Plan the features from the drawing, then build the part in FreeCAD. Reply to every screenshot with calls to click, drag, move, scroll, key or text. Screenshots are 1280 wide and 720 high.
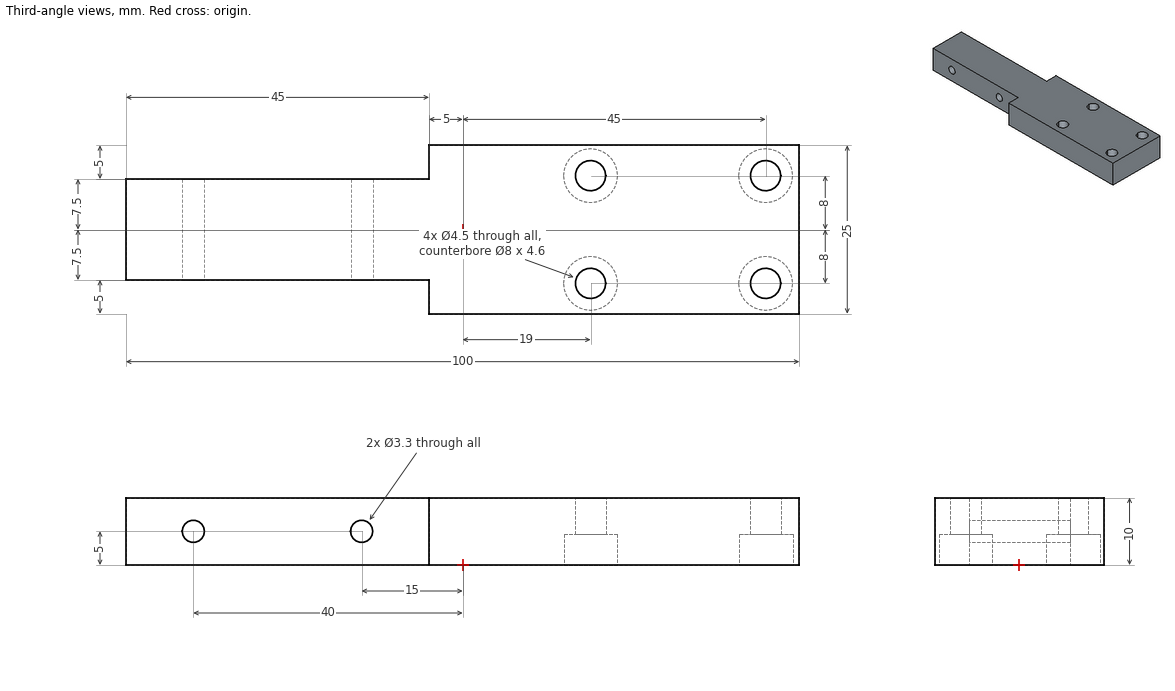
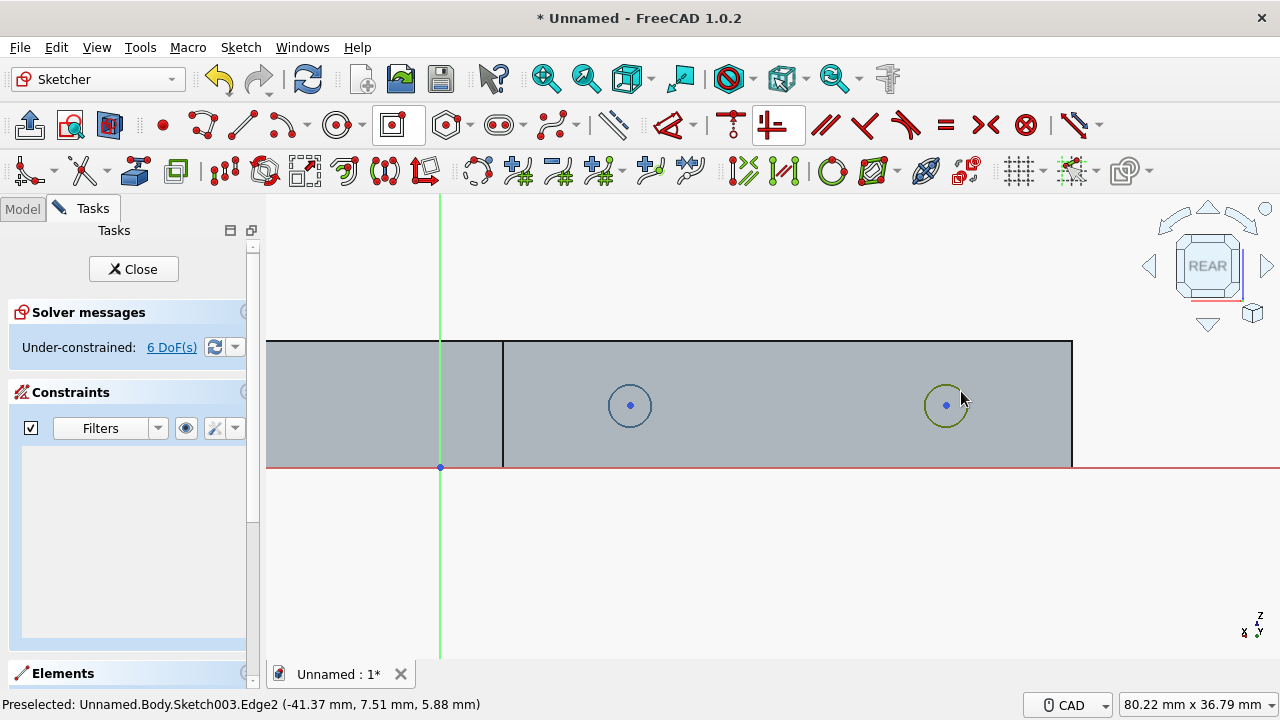
click(946, 126)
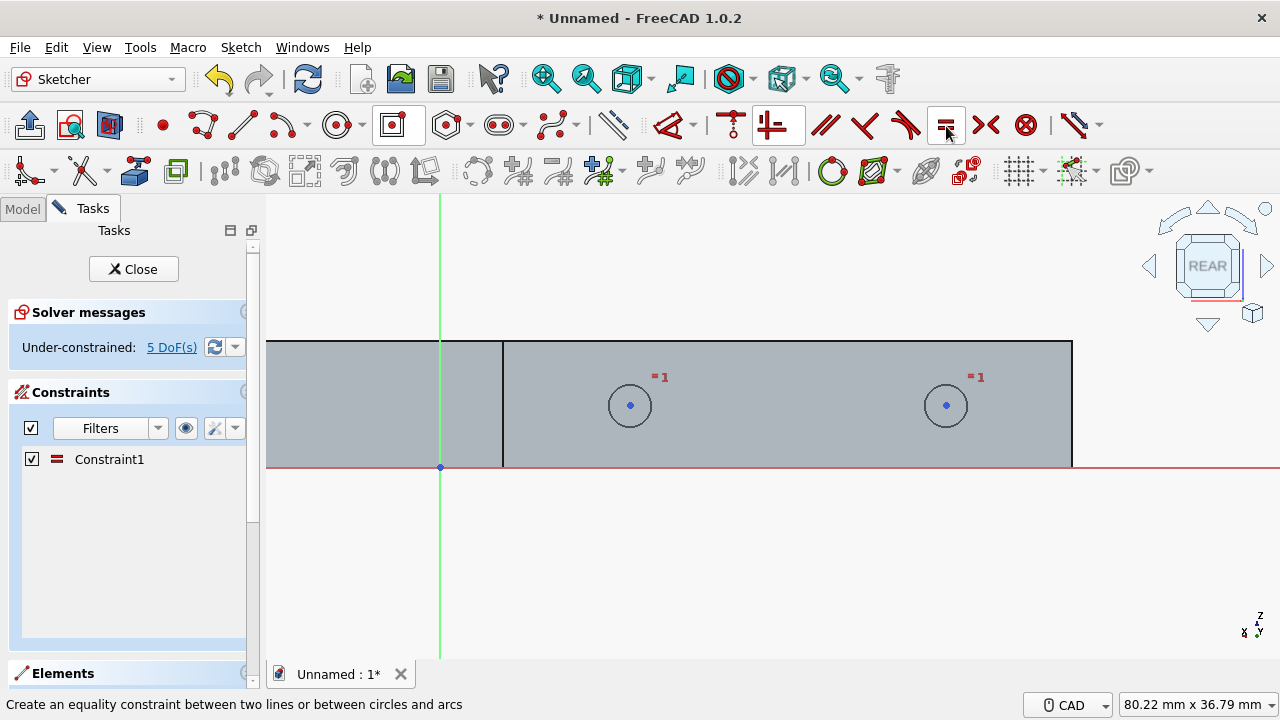
click(630, 406)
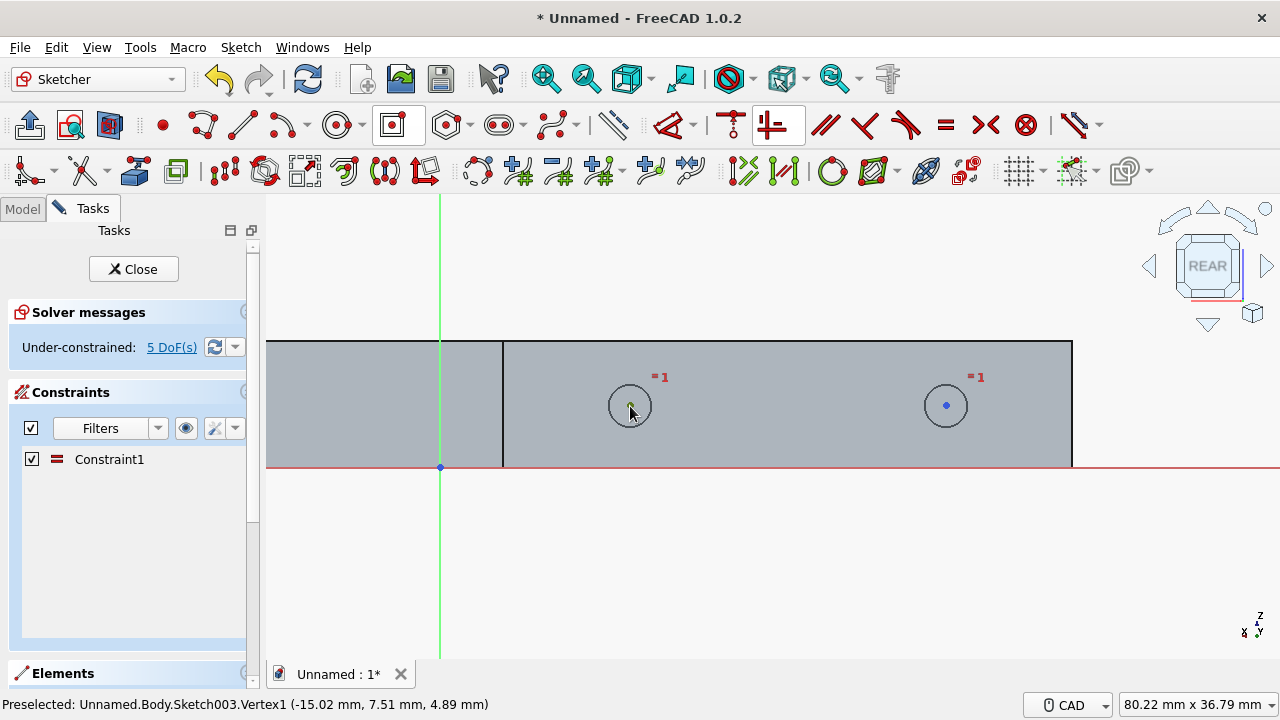
click(946, 406)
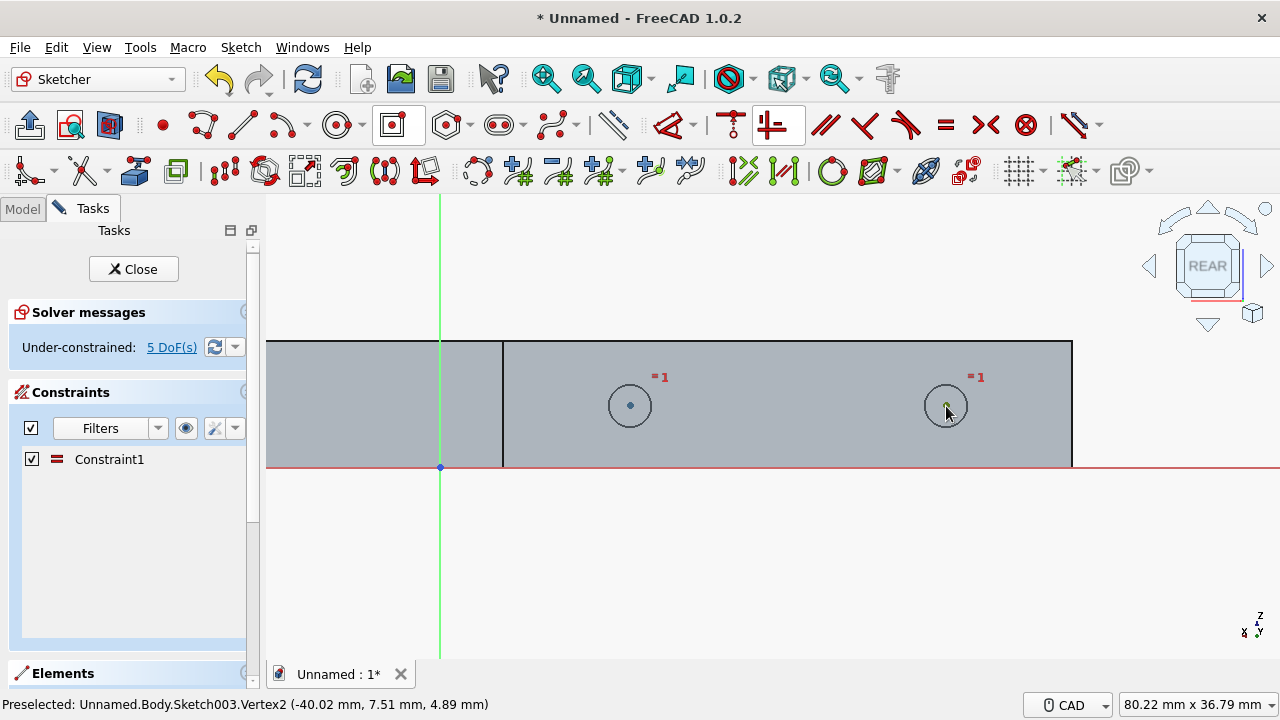
click(800, 126)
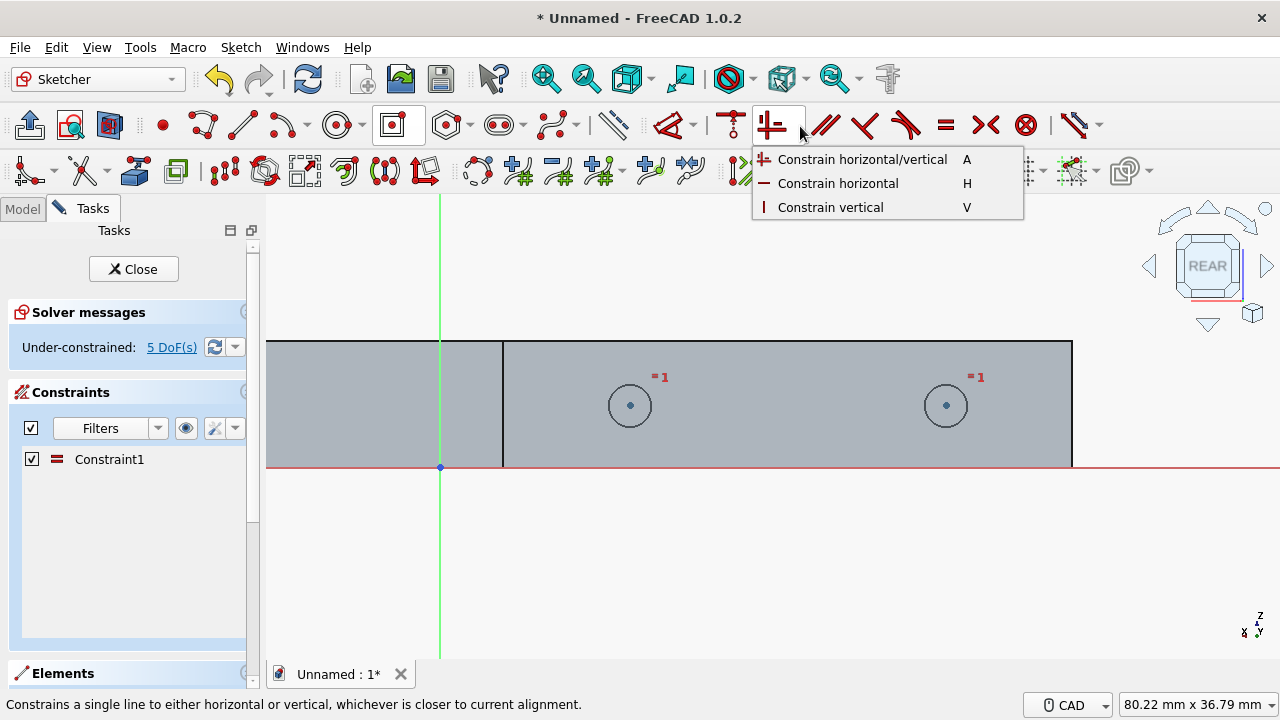
click(888, 183)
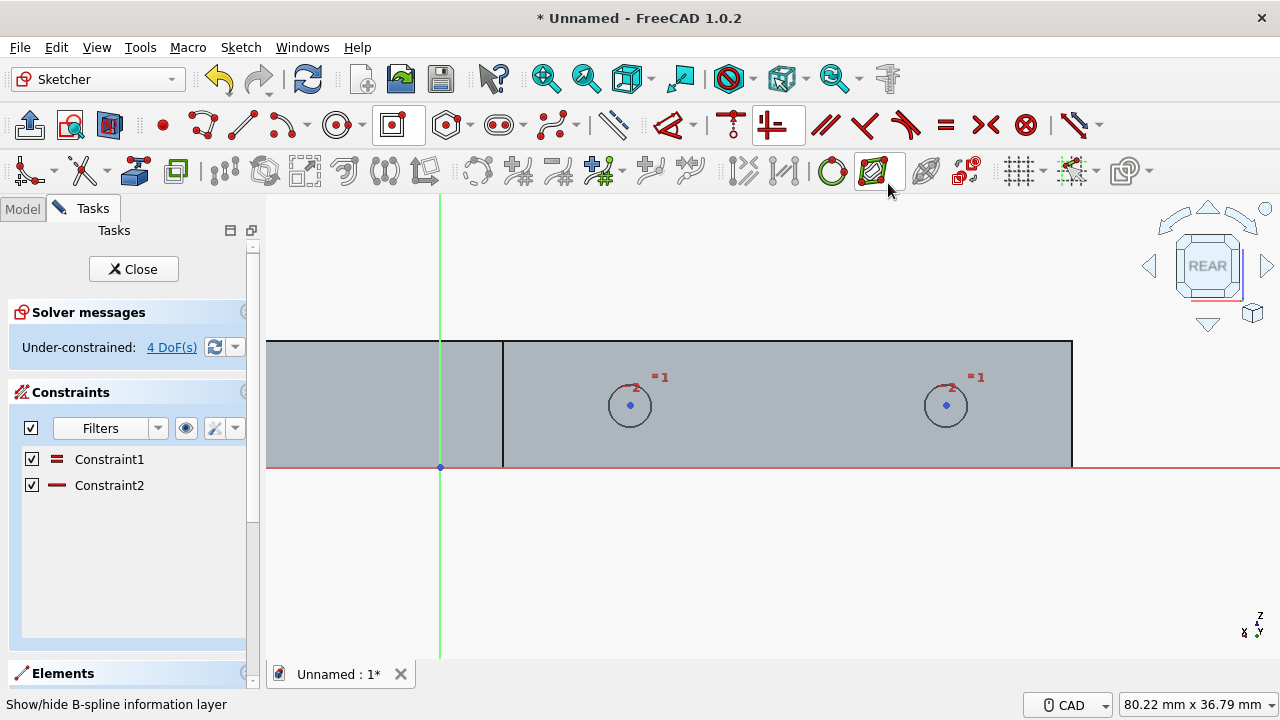
click(668, 126)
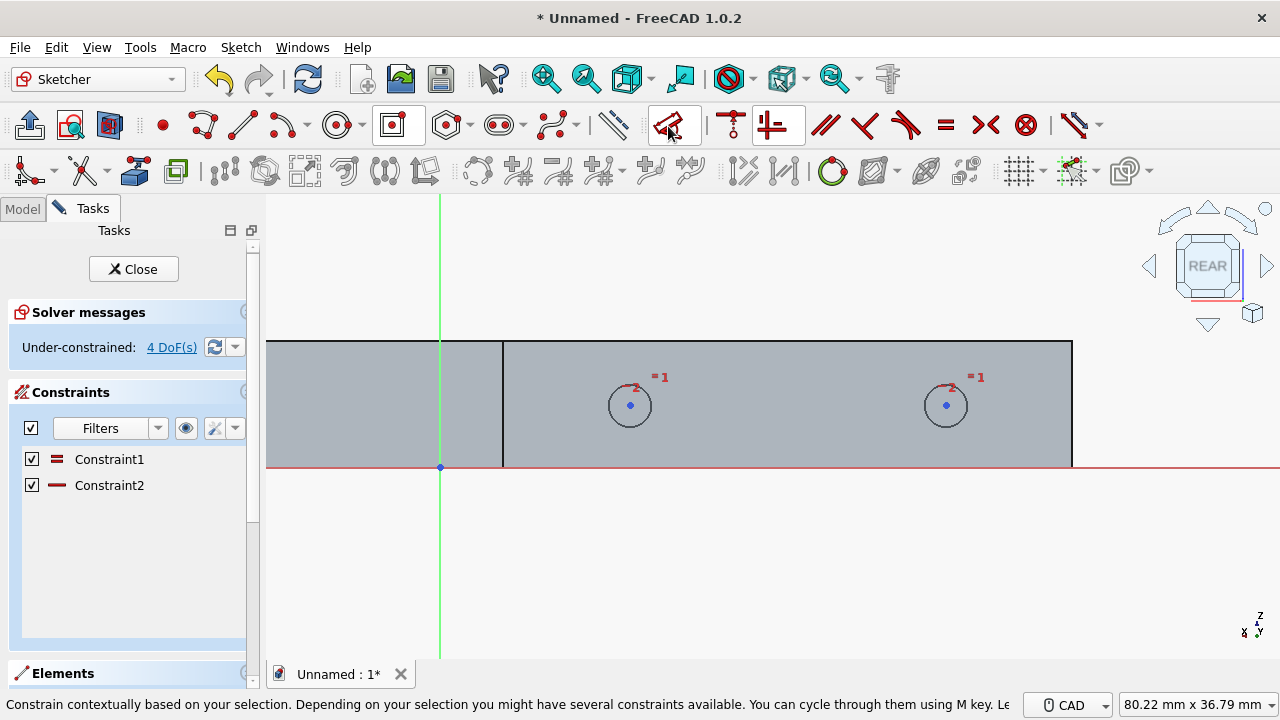
click(645, 391)
click(668, 368)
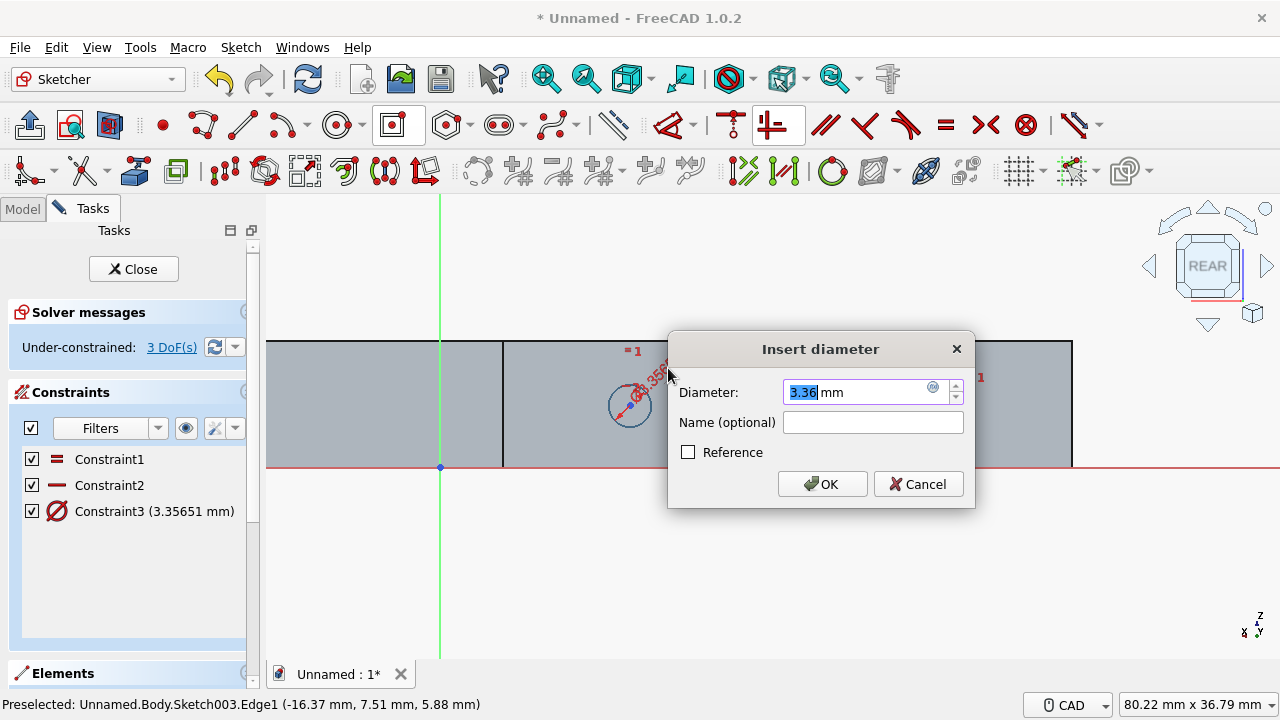
text(3.3)
key(Return)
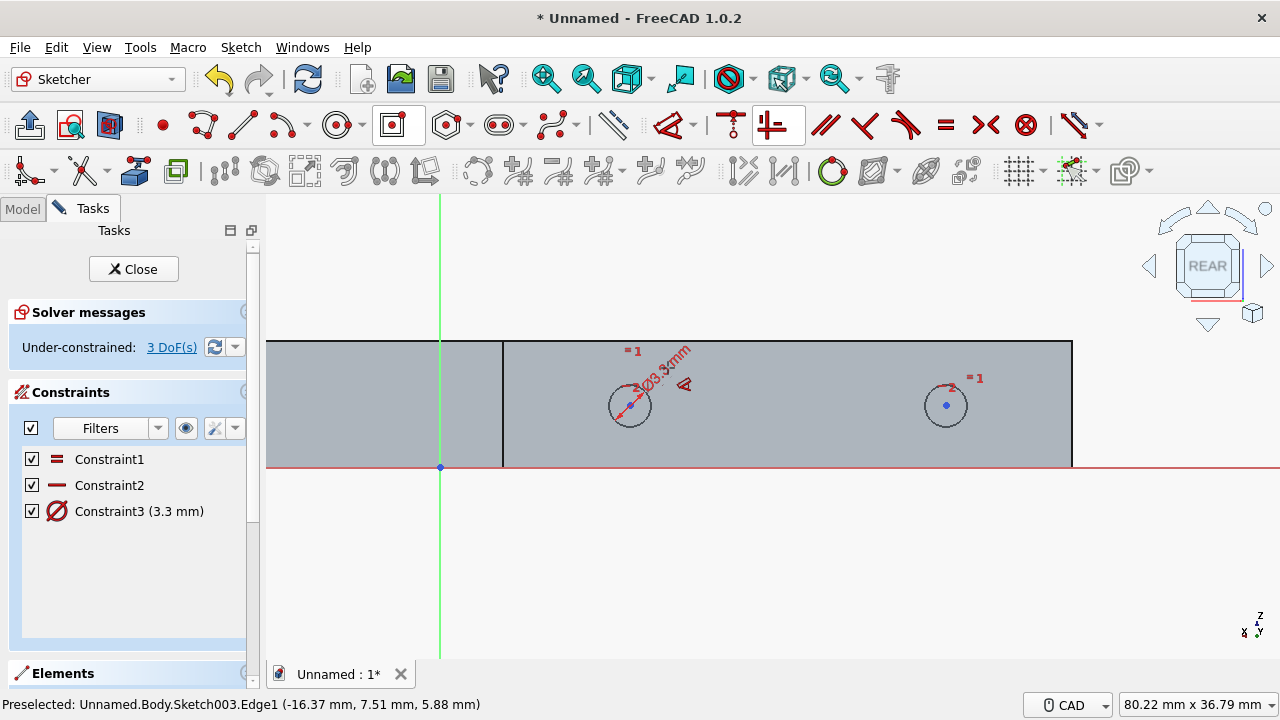
click(630, 406)
click(406, 437)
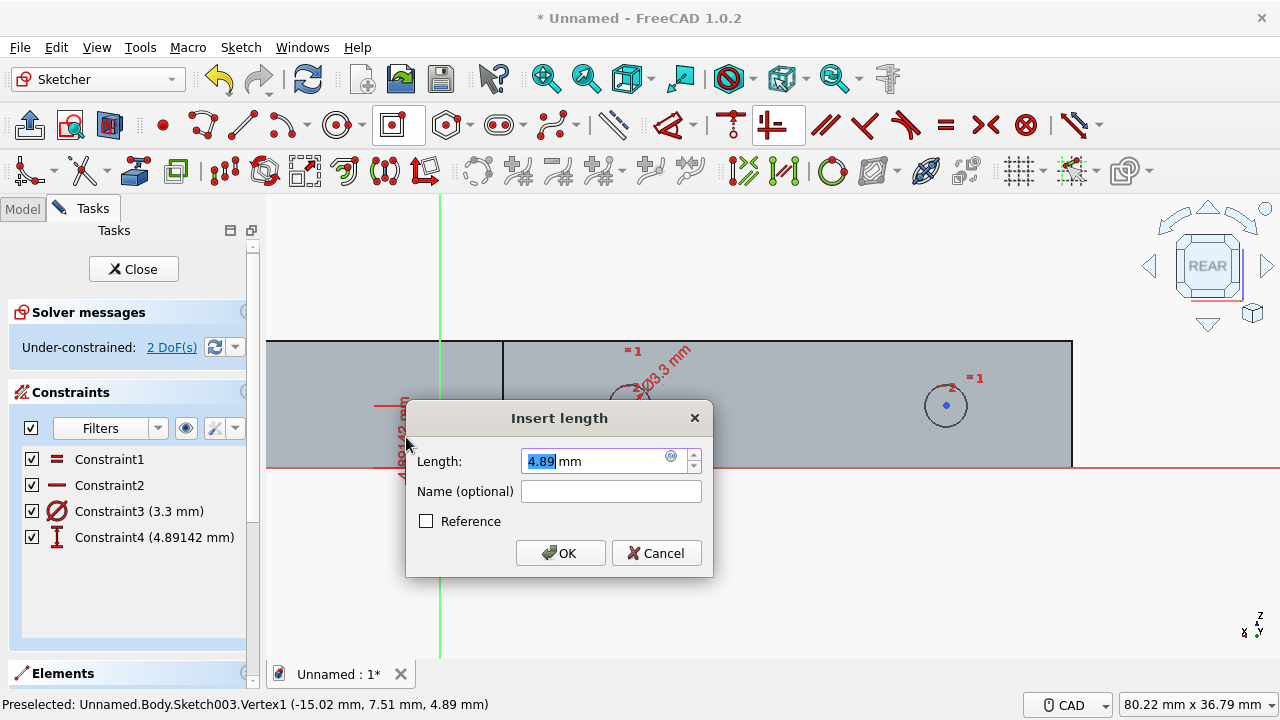
text(5)
key(Return)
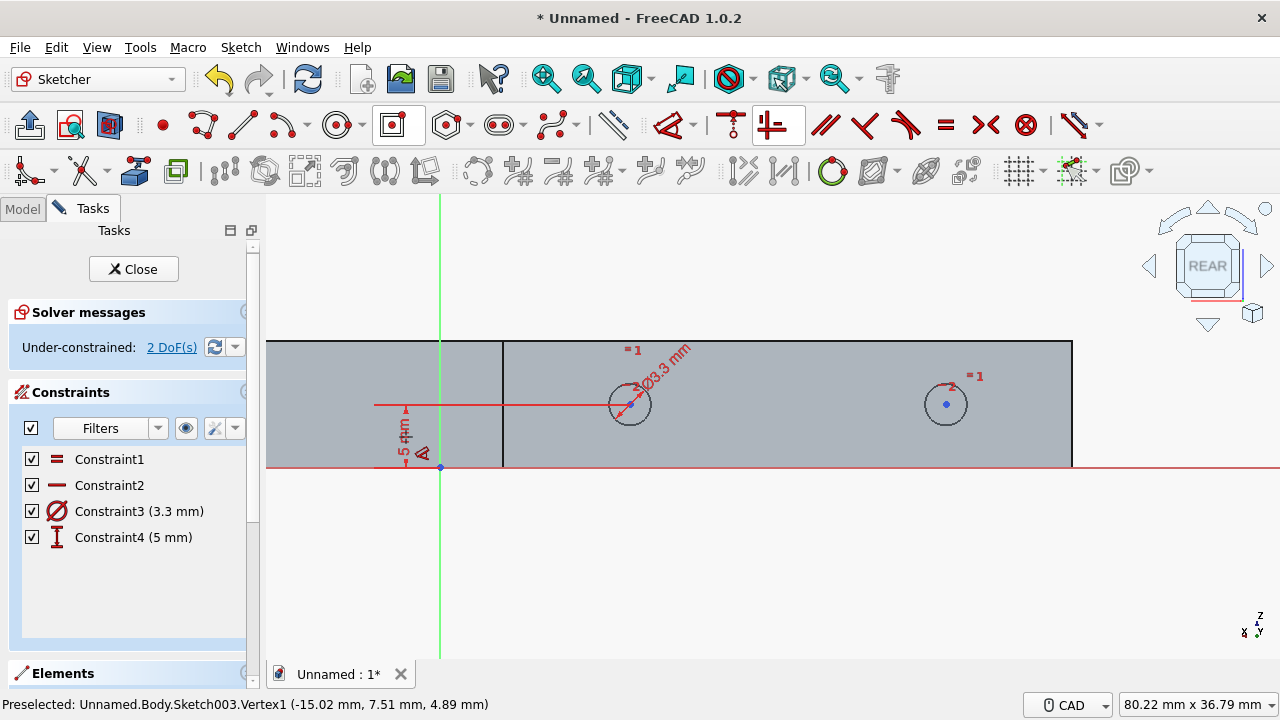
click(630, 405)
click(535, 502)